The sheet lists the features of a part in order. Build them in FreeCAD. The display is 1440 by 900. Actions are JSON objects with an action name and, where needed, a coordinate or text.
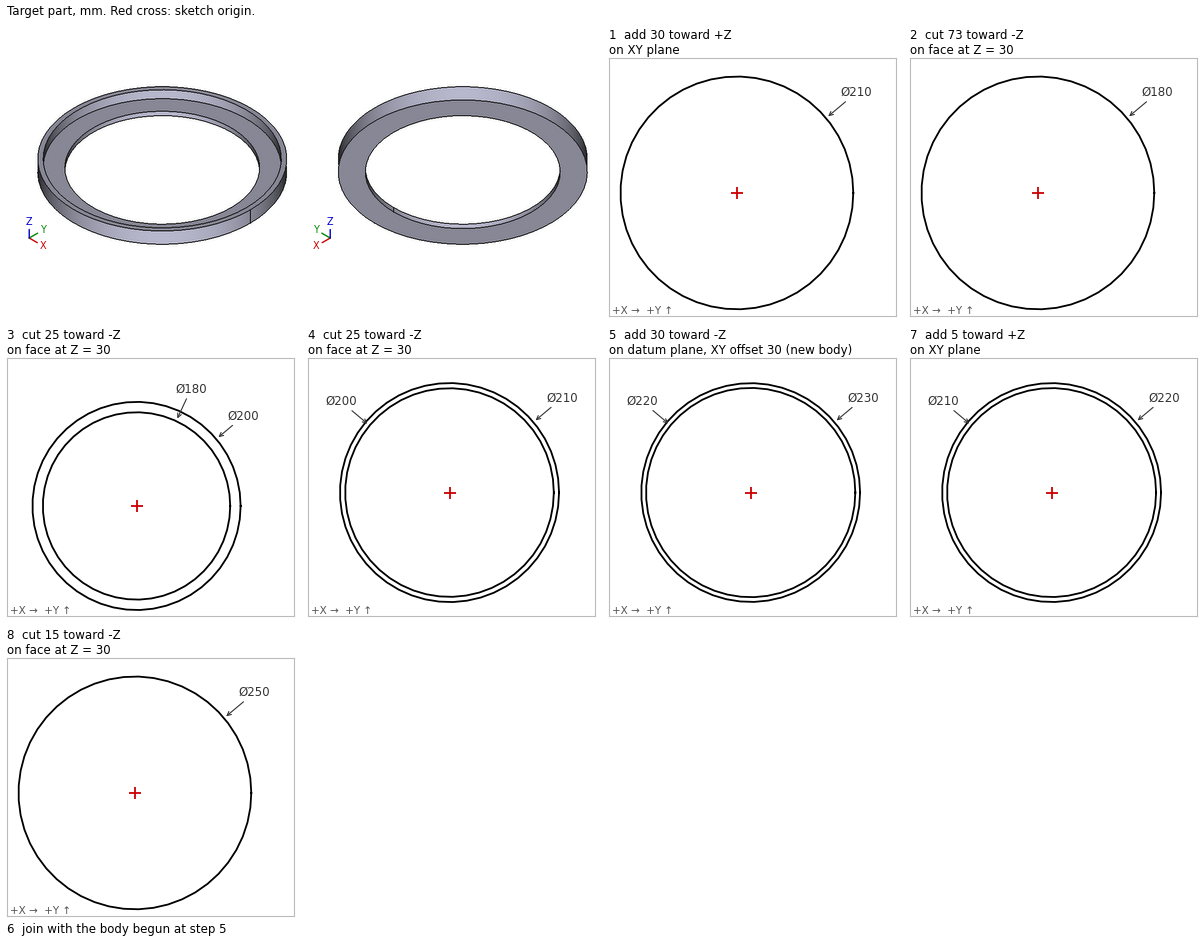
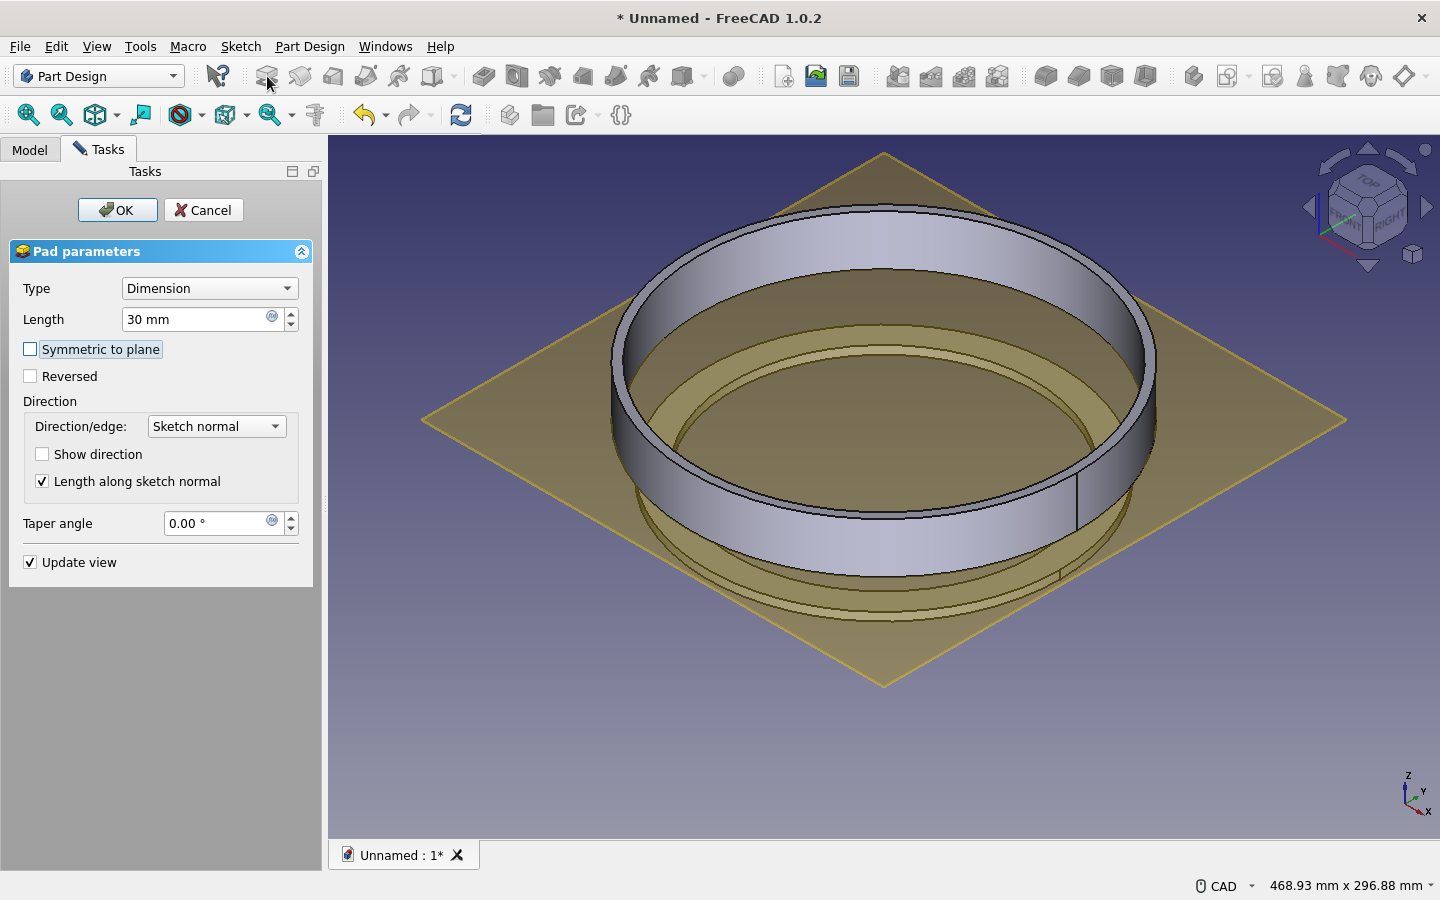
{"action": "left_click", "coordinate": [31, 376]}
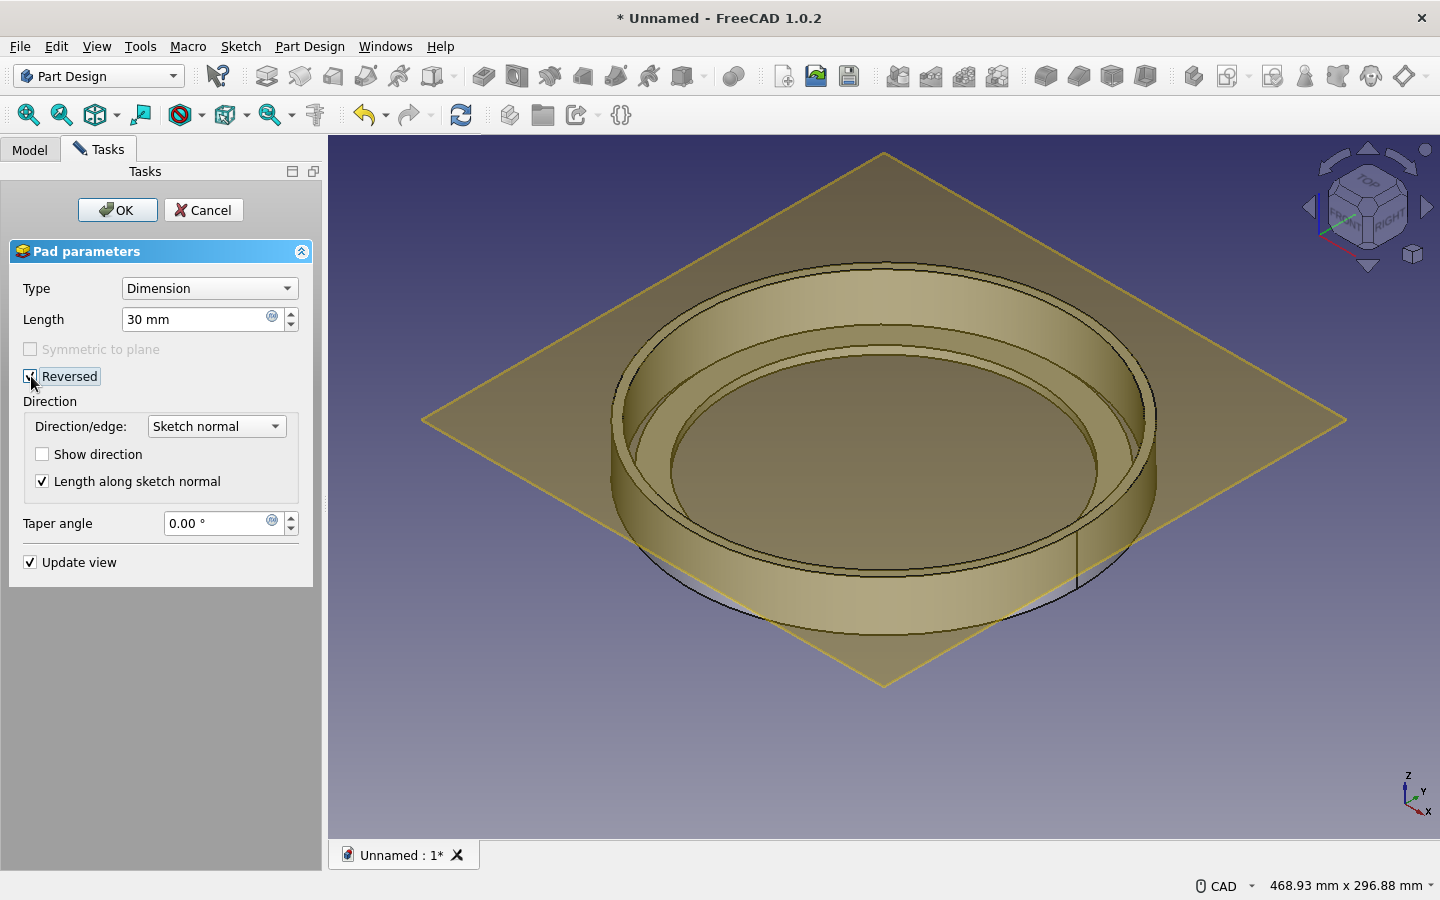
{"action": "left_click", "coordinate": [118, 210]}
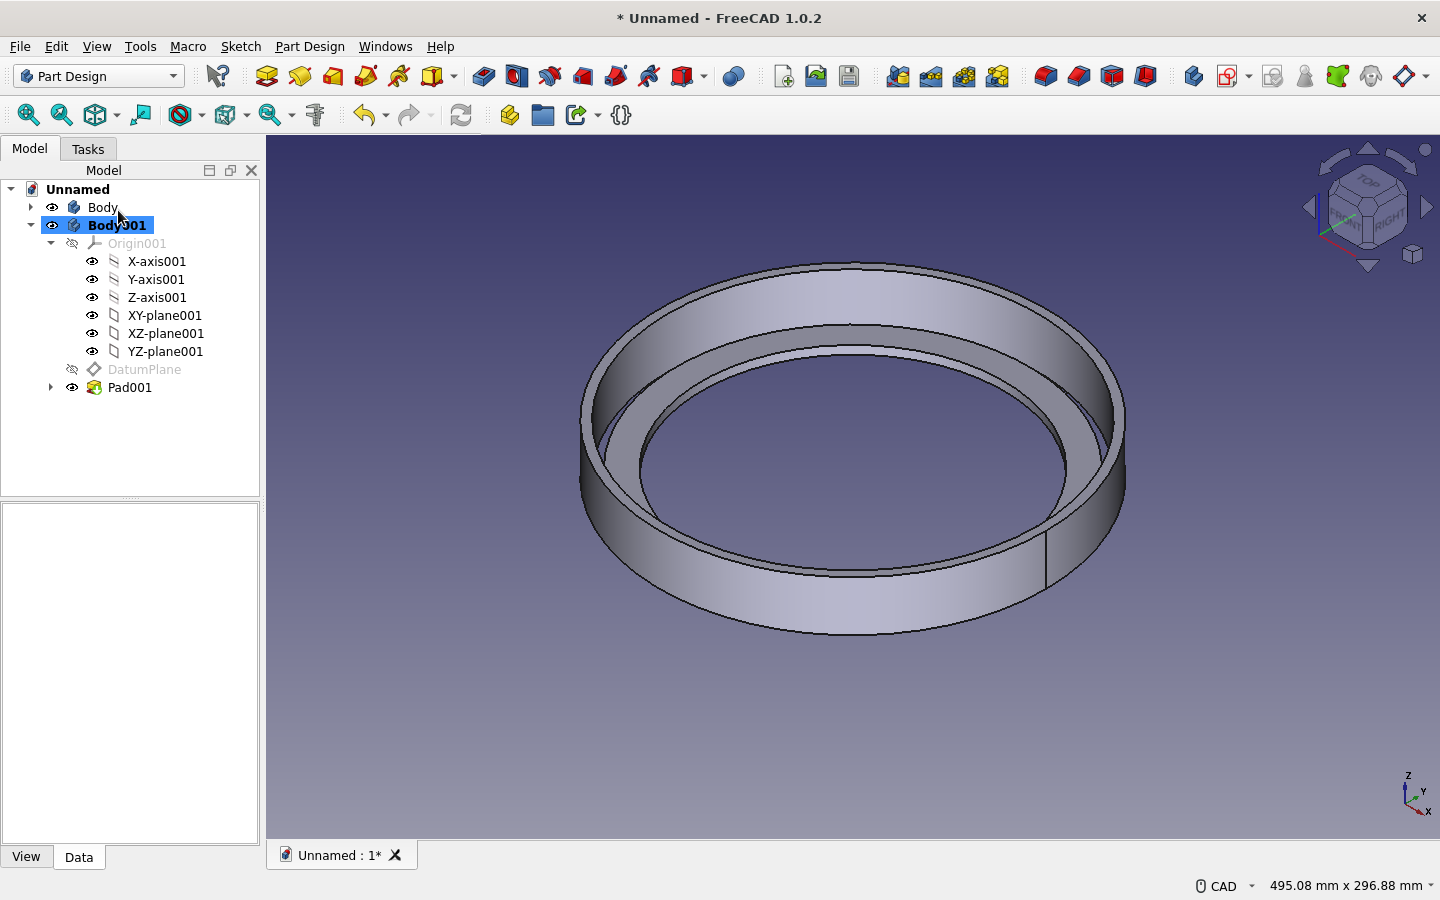
{"action": "double_click", "coordinate": [97, 207]}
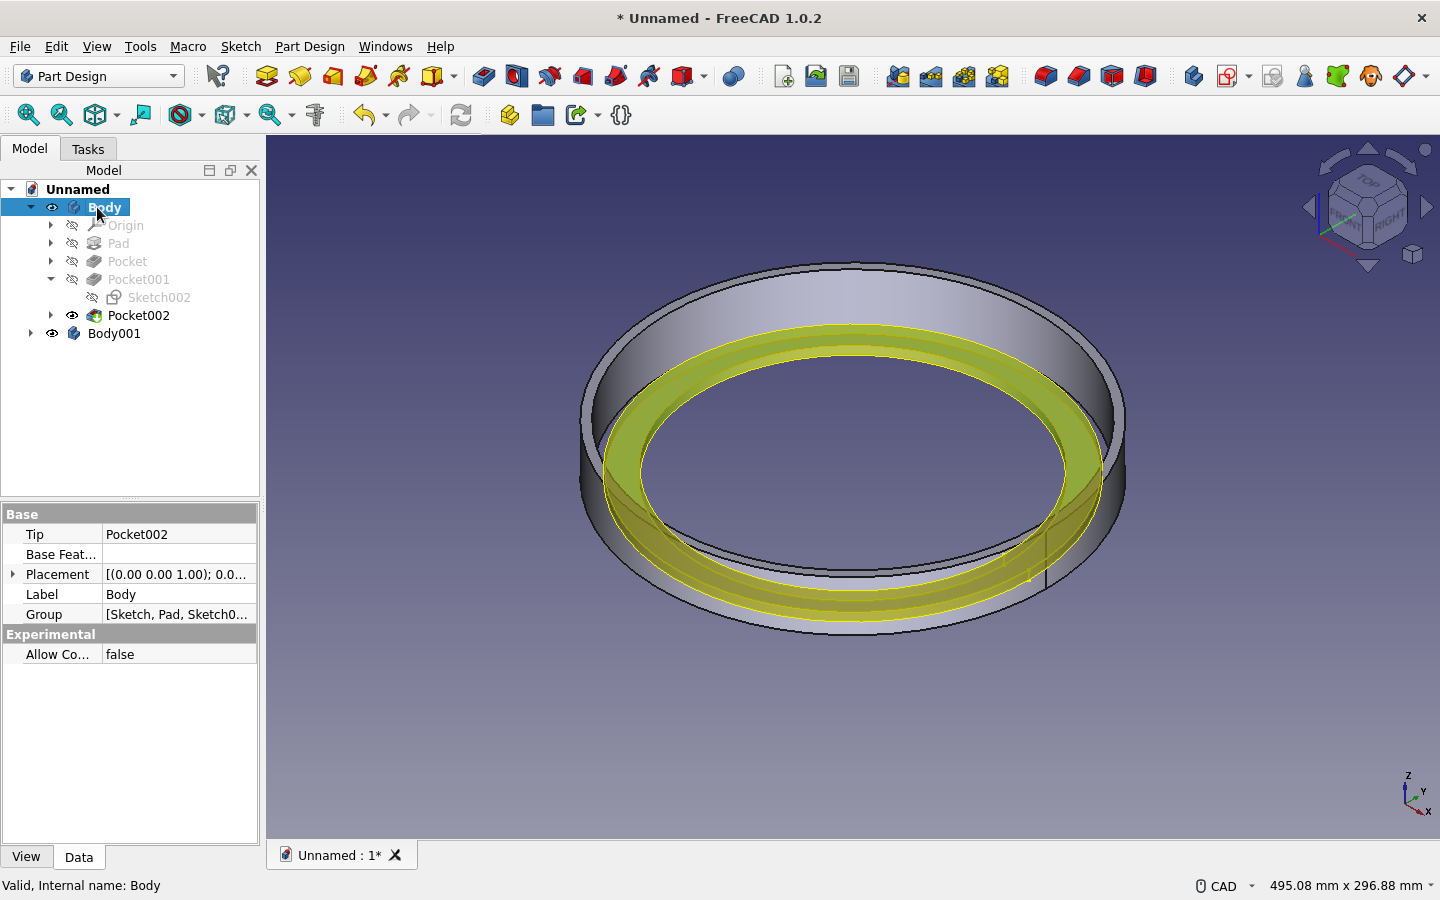
{"action": "left_click", "coordinate": [97, 207]}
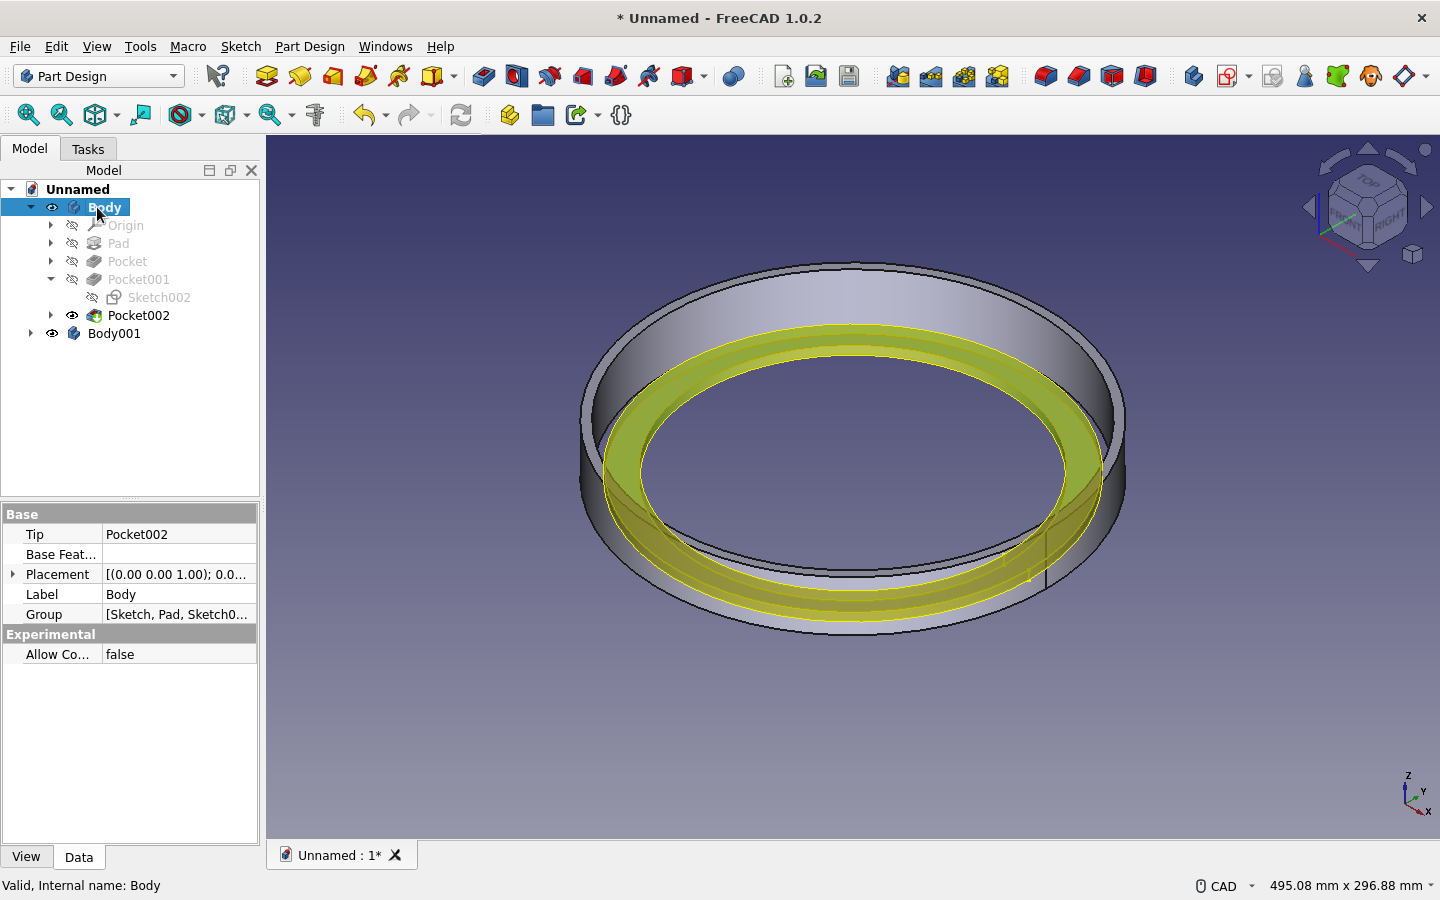
{"action": "left_click", "coordinate": [148, 654]}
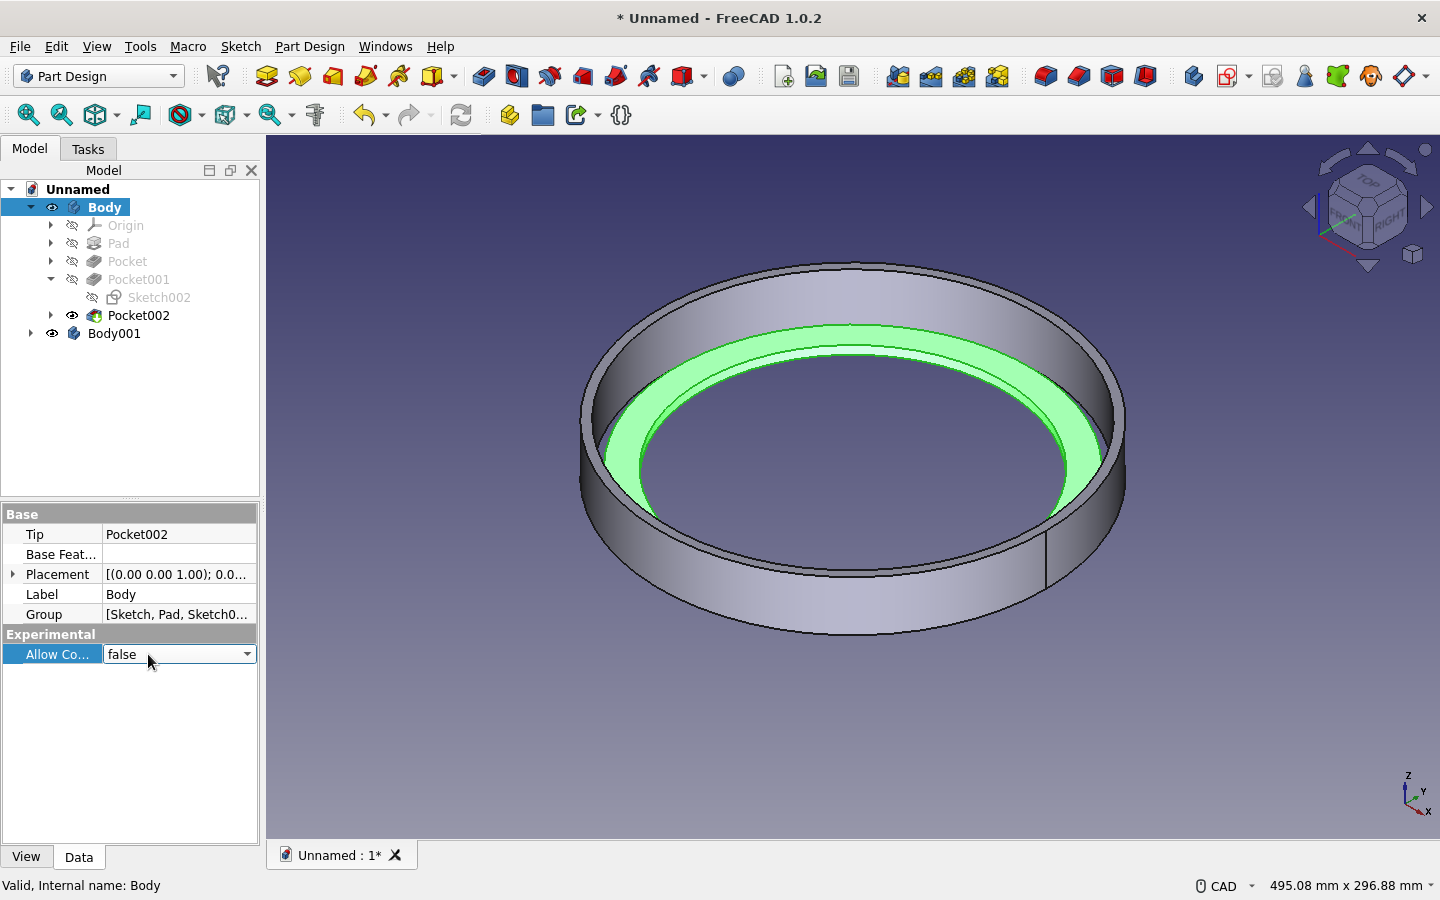
{"action": "left_click", "coordinate": [148, 654]}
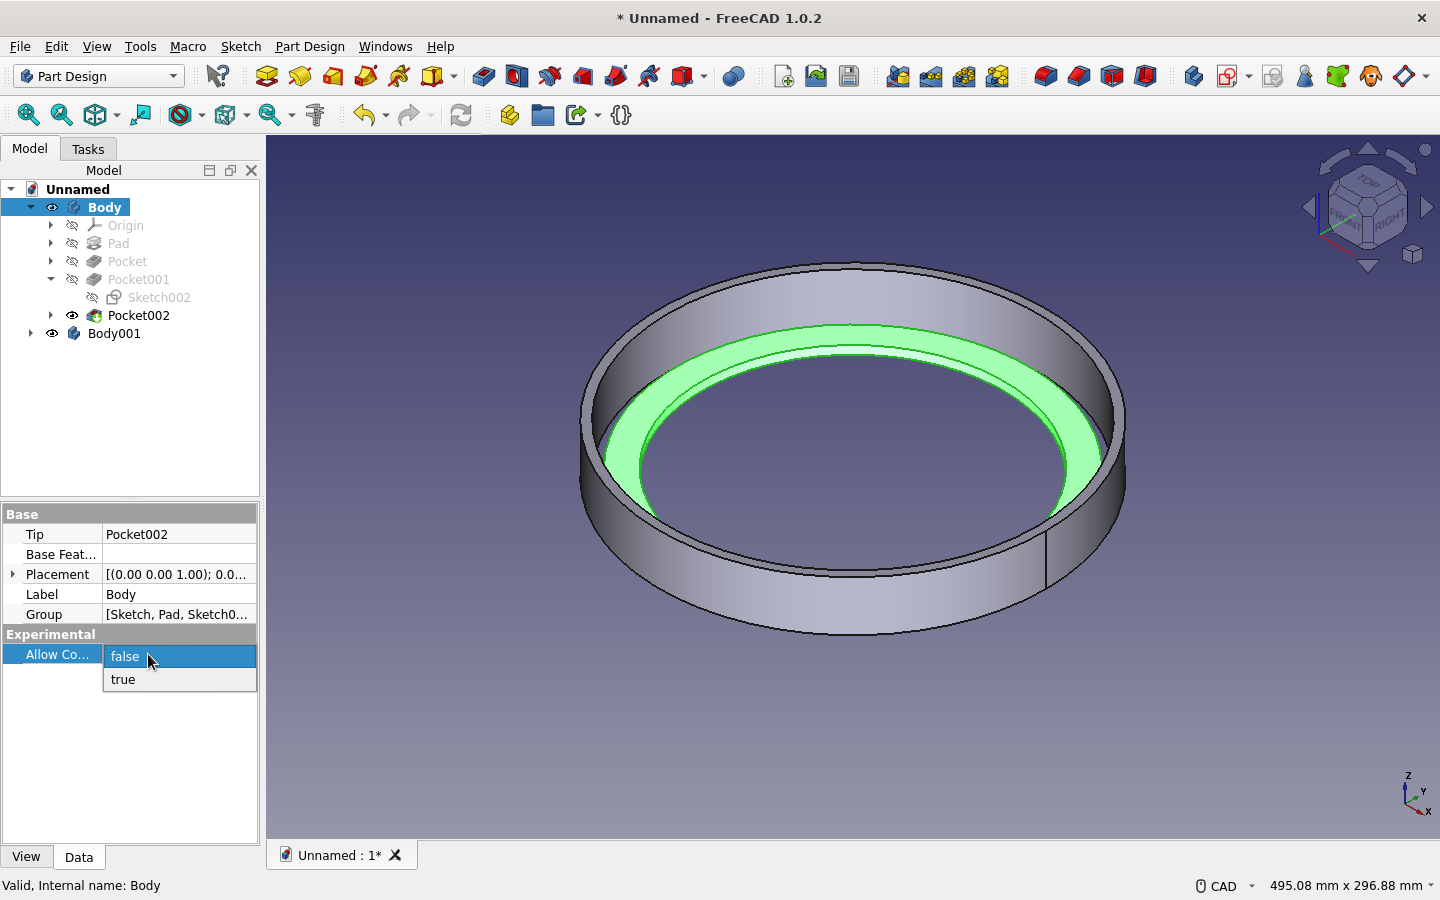
{"action": "left_click", "coordinate": [178, 680]}
{"action": "key", "text": "Return"}